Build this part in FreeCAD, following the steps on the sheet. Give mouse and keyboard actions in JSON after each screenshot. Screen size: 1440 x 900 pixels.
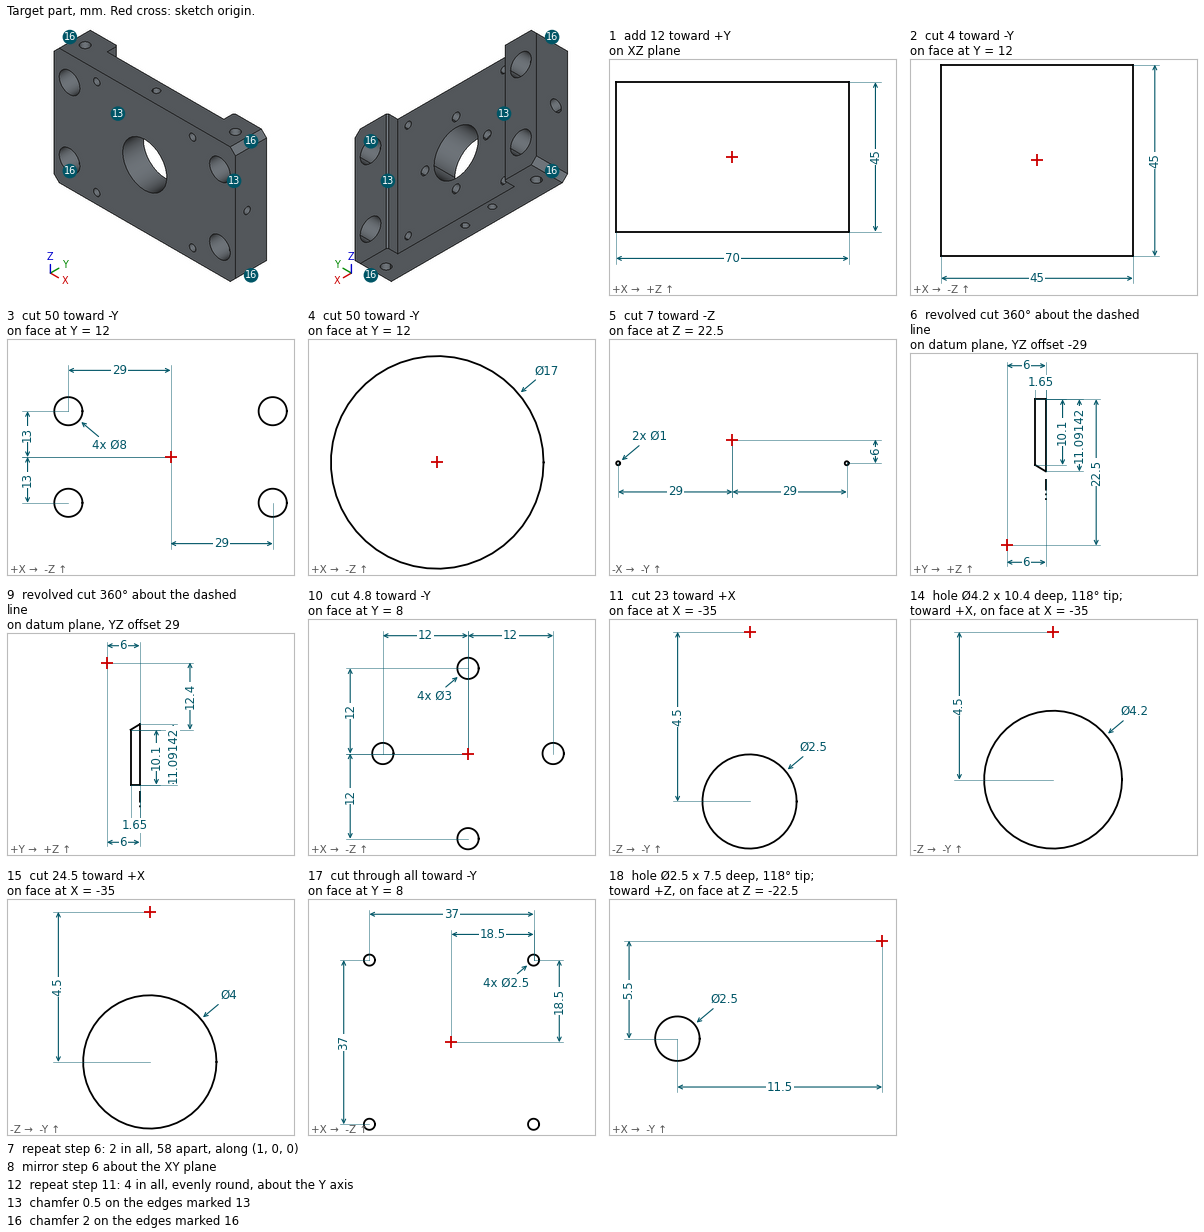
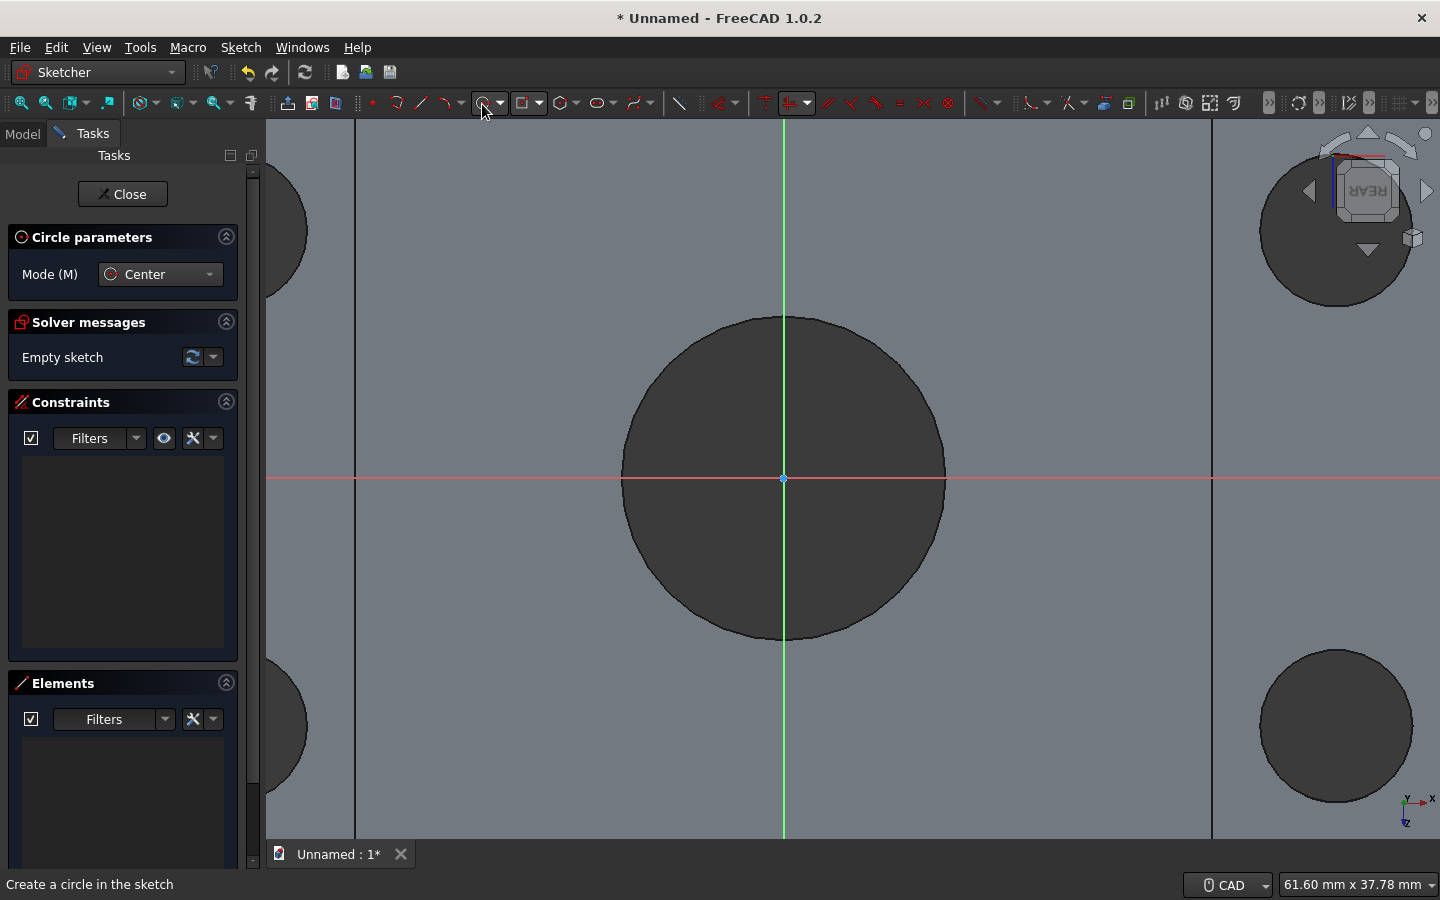
{"action": "left_click", "coordinate": [784, 250]}
{"action": "mouse_move", "coordinate": [804, 229]}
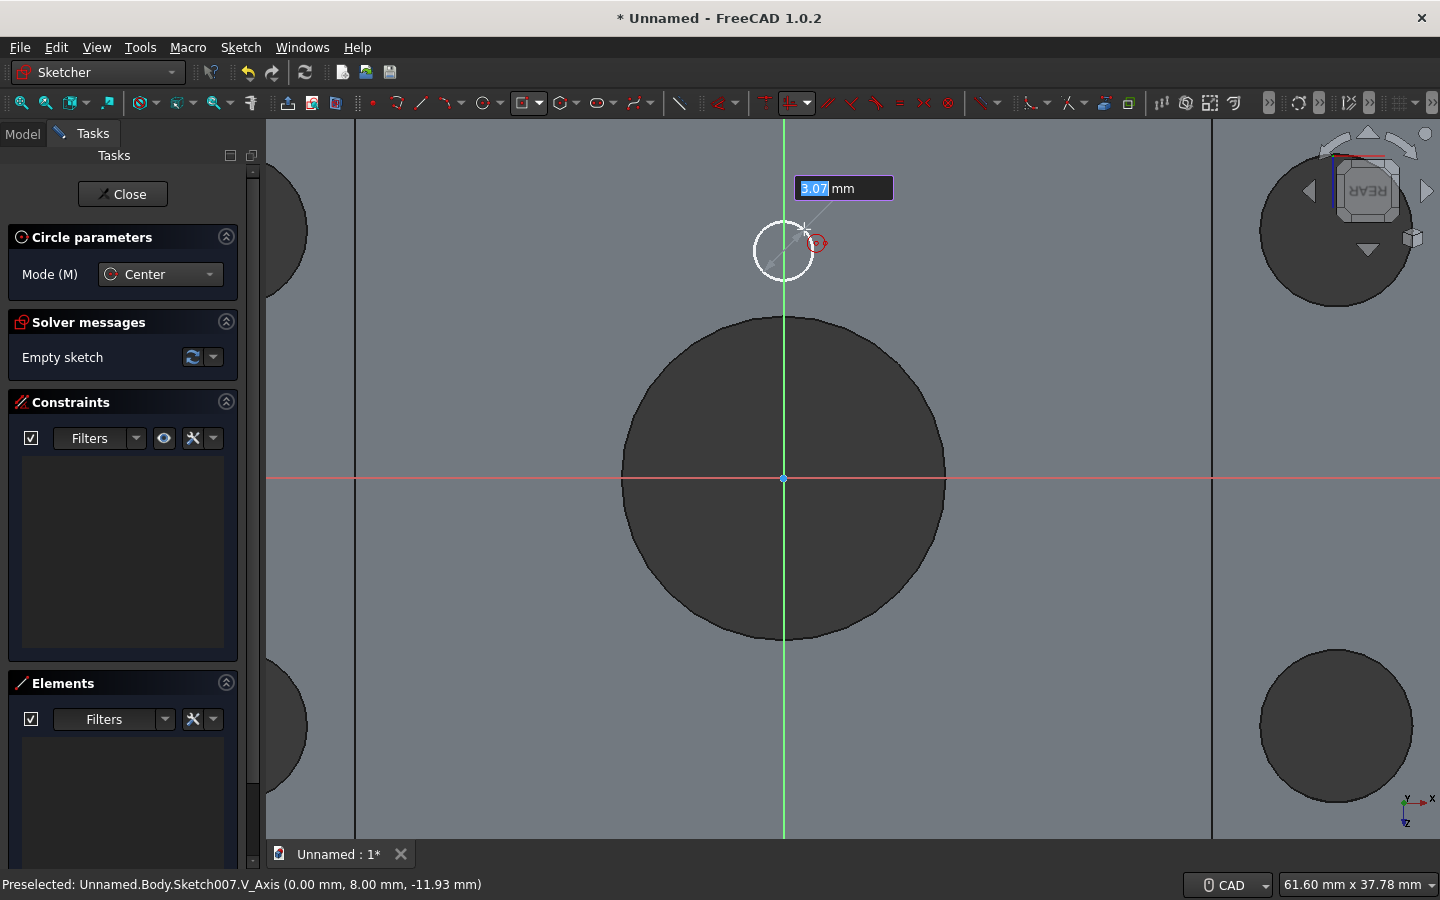
{"action": "type", "text": "3"}
{"action": "key", "text": "Return"}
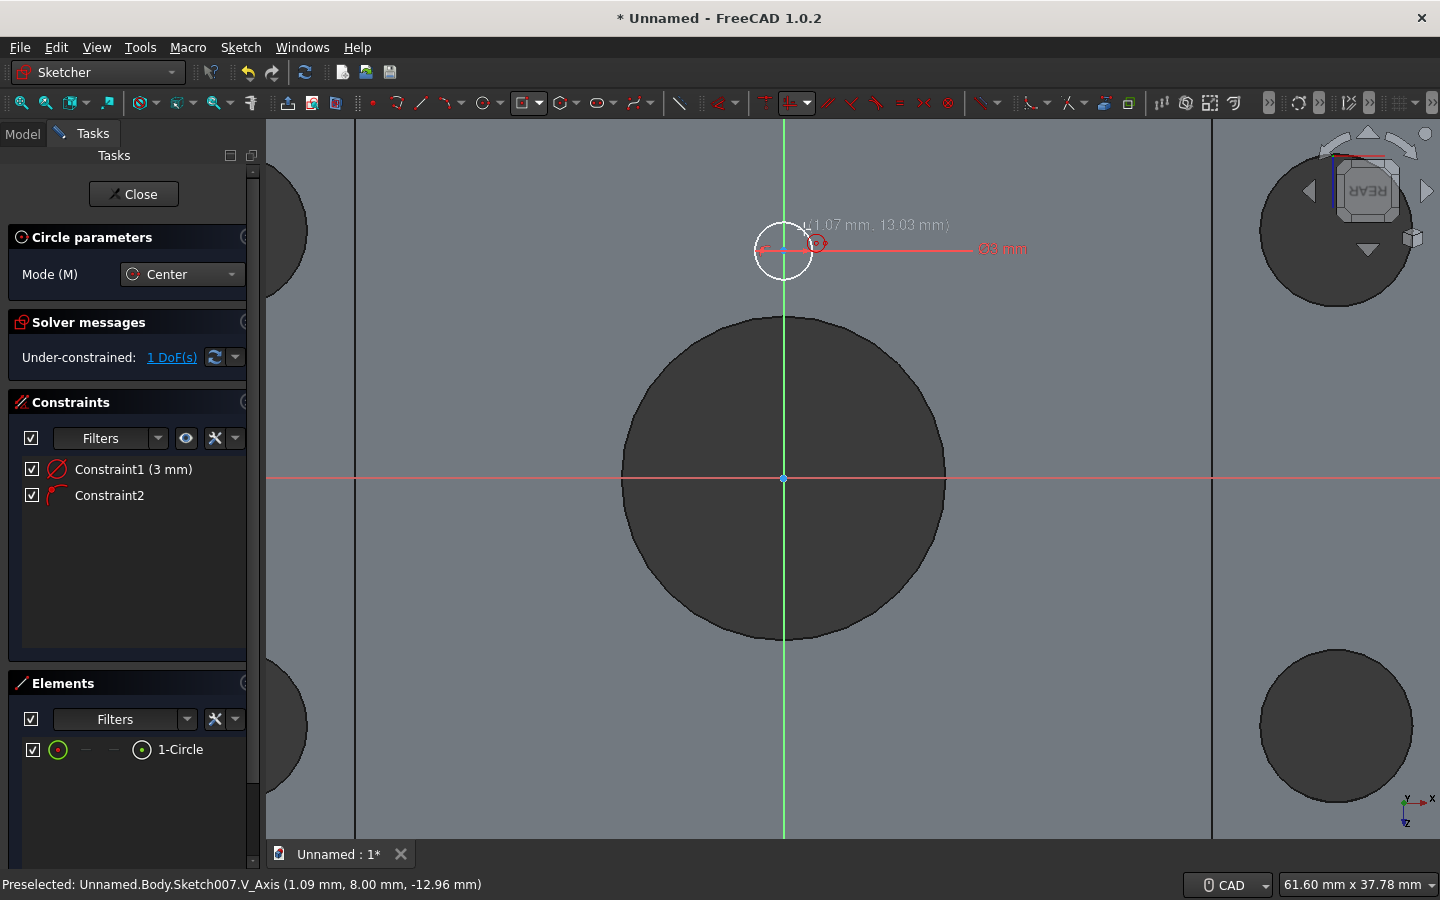
{"action": "left_click", "coordinate": [1012, 478]}
{"action": "mouse_move", "coordinate": [1033, 458]}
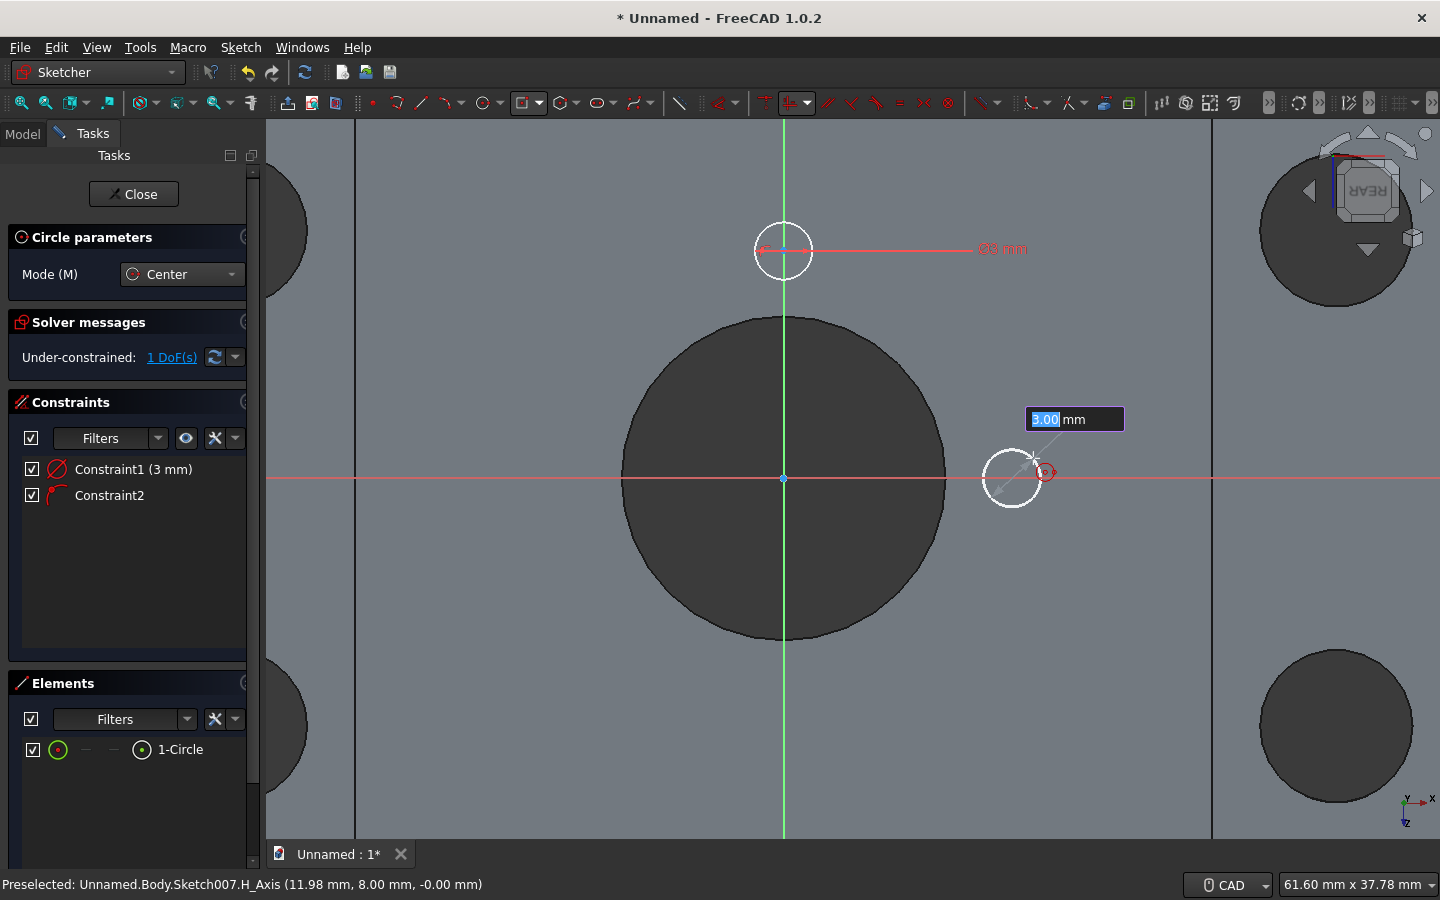
{"action": "type", "text": "3"}
{"action": "key", "text": "Return"}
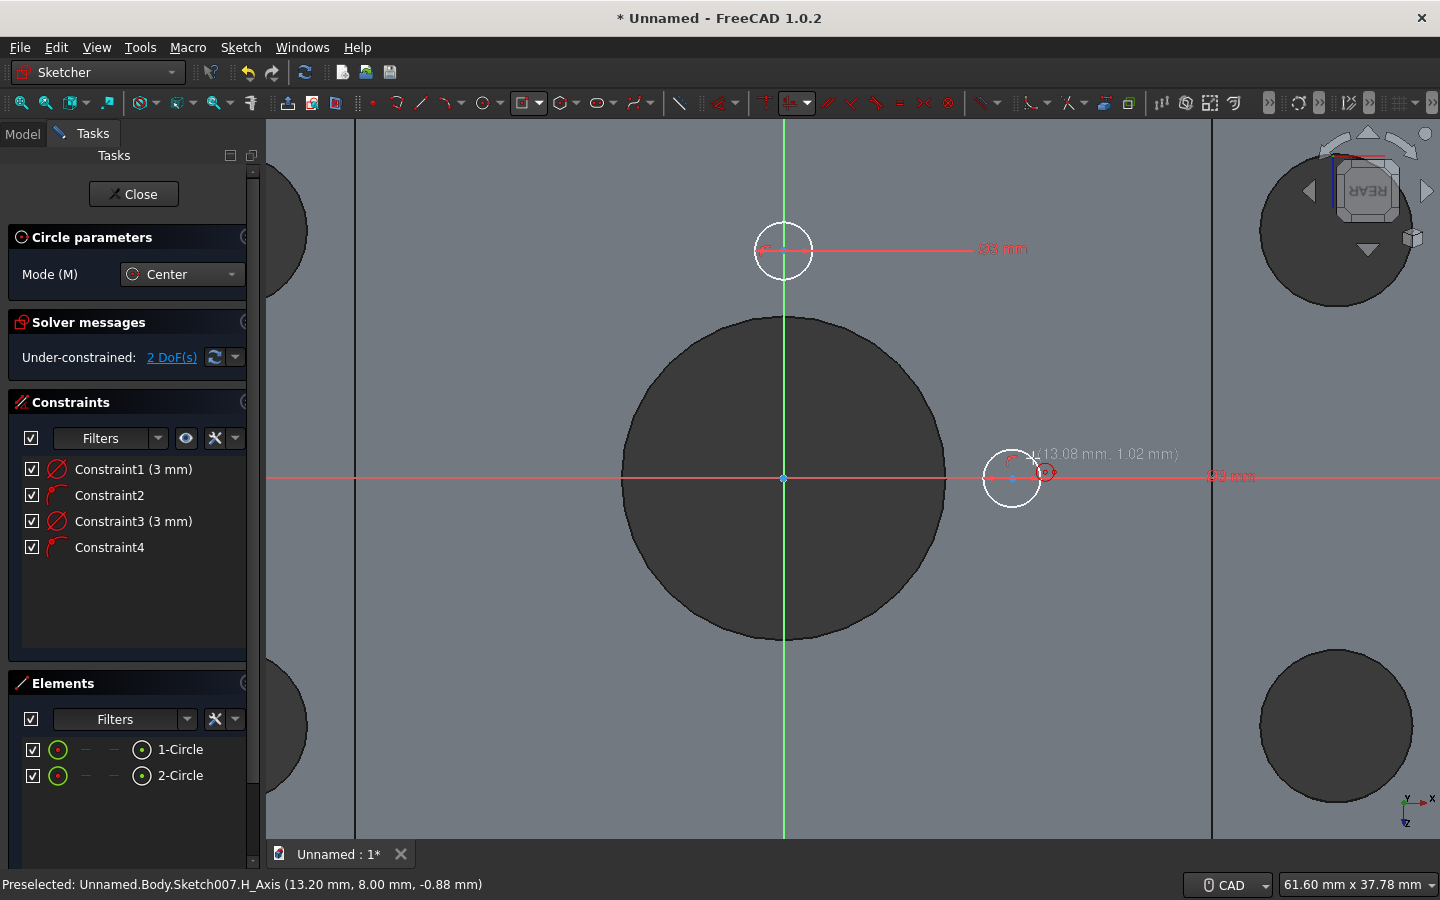
{"action": "left_click", "coordinate": [784, 707]}
{"action": "mouse_move", "coordinate": [804, 687]}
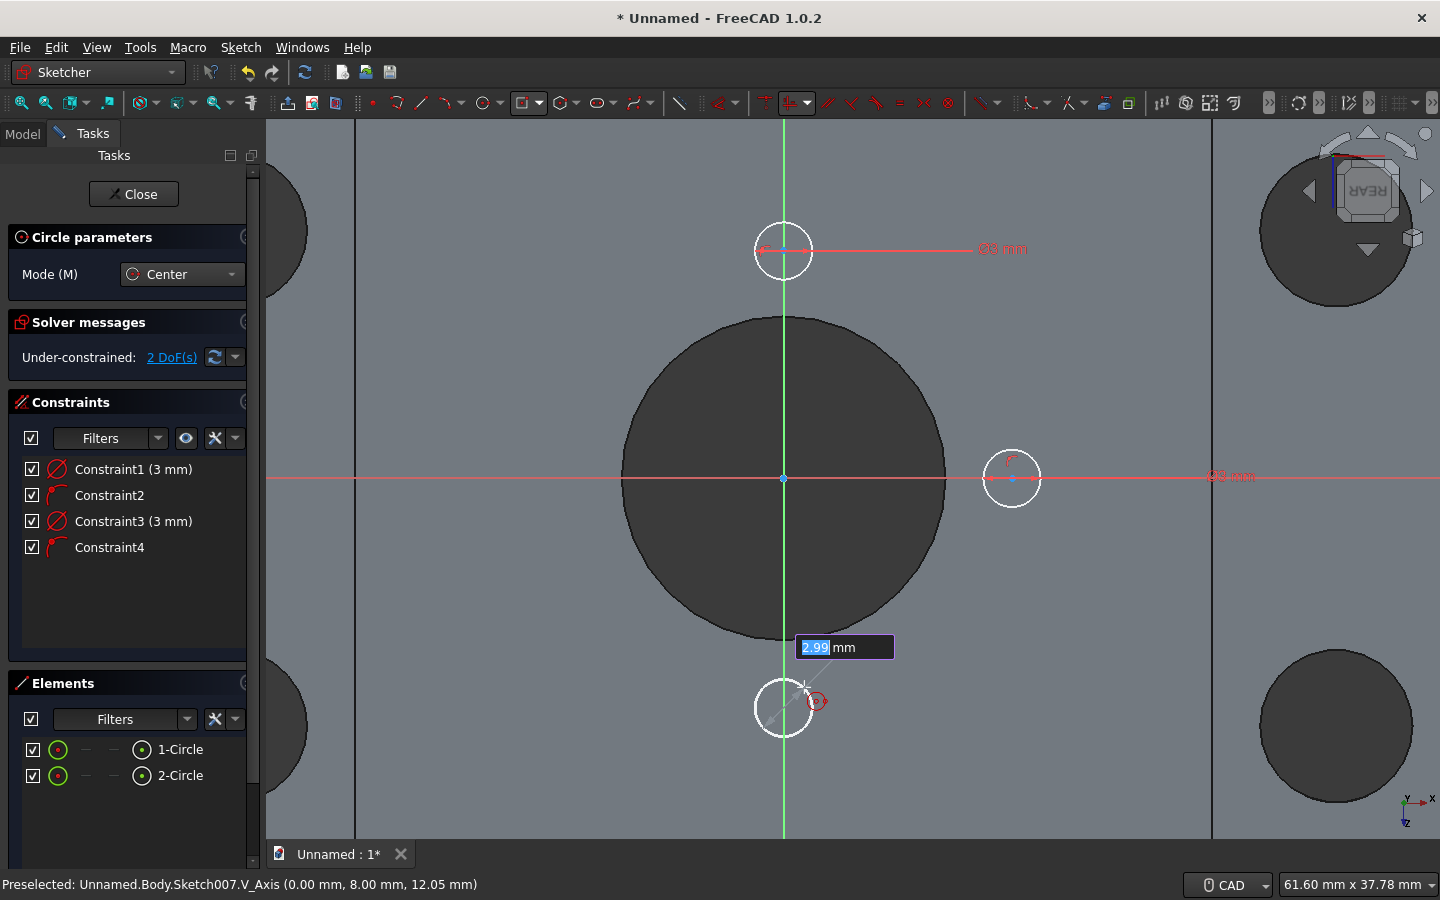
{"action": "type", "text": "3"}
{"action": "key", "text": "Return"}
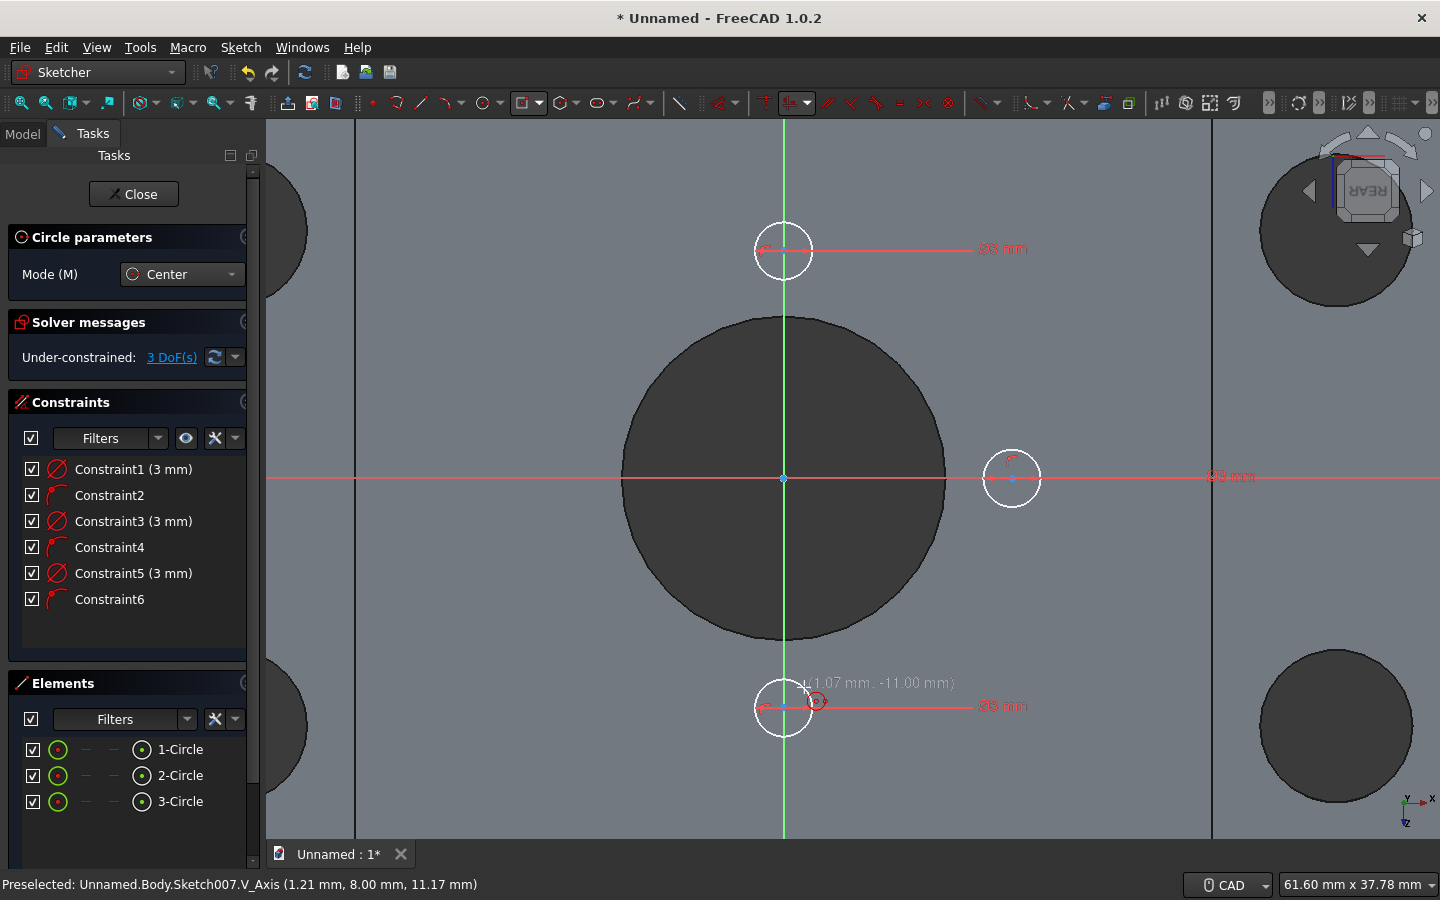
{"action": "left_click", "coordinate": [555, 478]}
{"action": "mouse_move", "coordinate": [575, 458]}